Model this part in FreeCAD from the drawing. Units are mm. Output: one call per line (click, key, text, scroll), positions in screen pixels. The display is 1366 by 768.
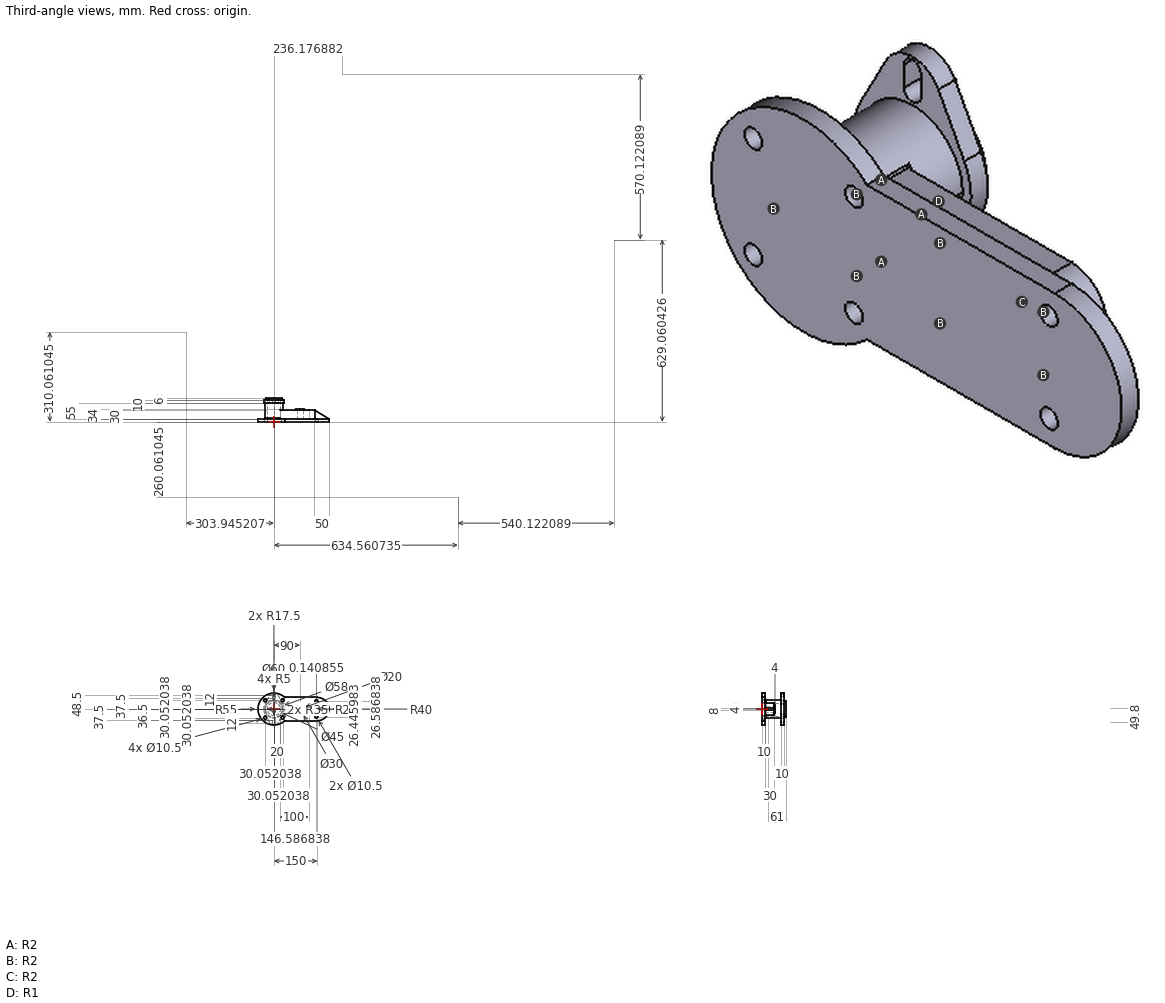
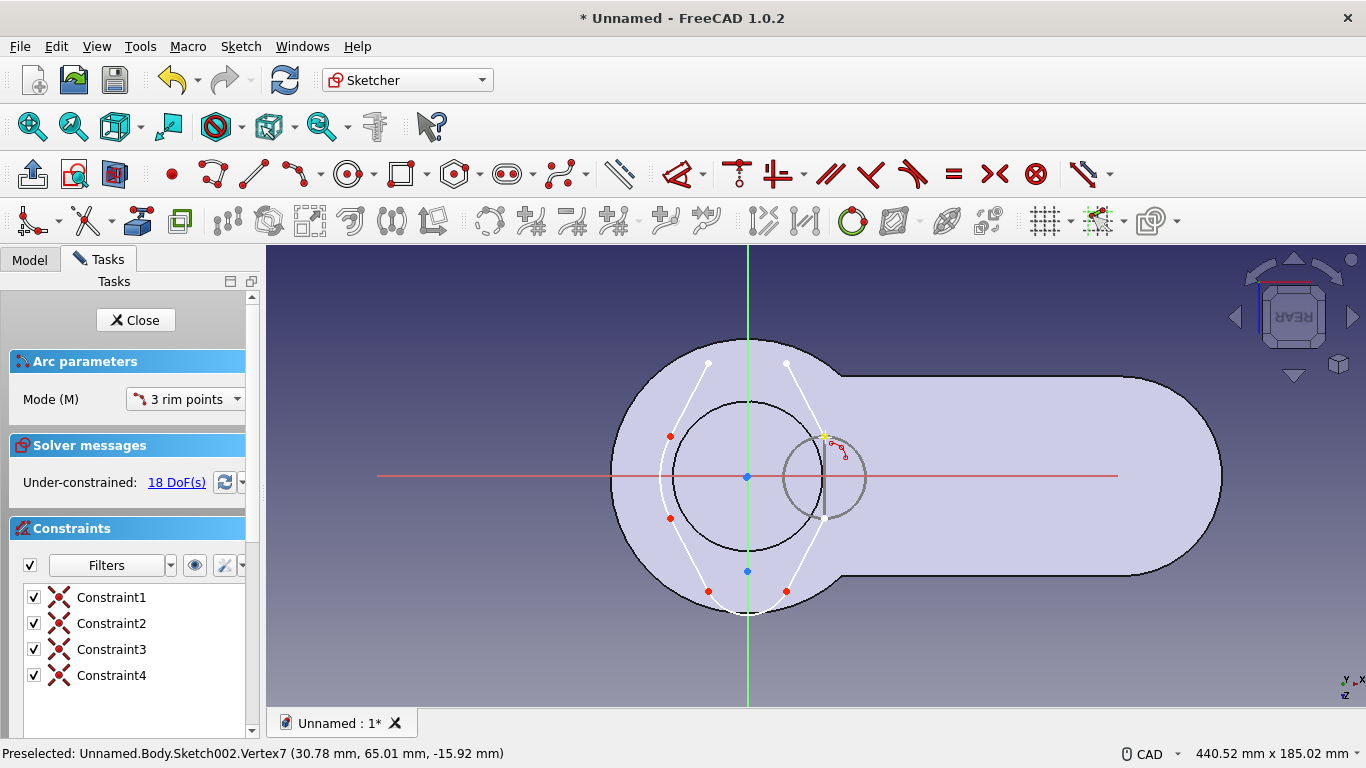
scroll(835, 468, up, 4)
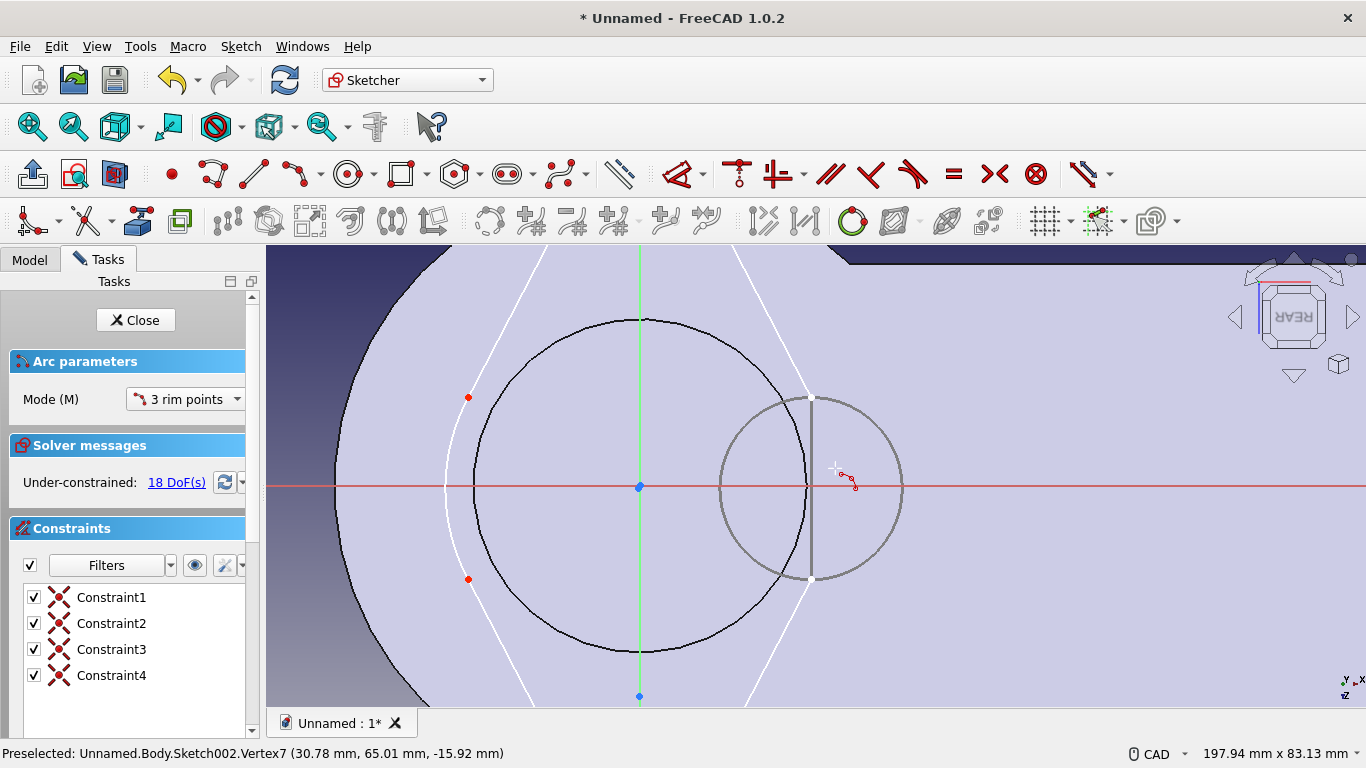
click(834, 467)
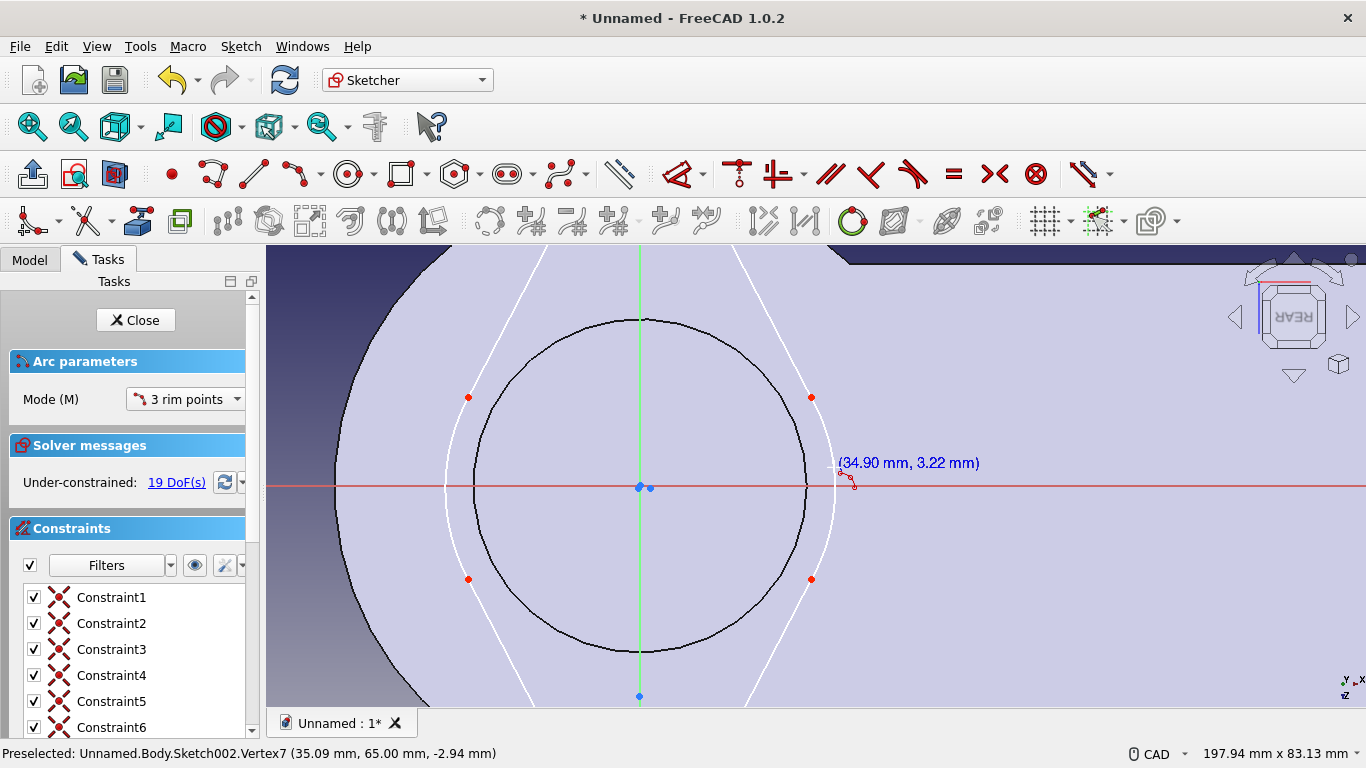
scroll(835, 468, down, 4)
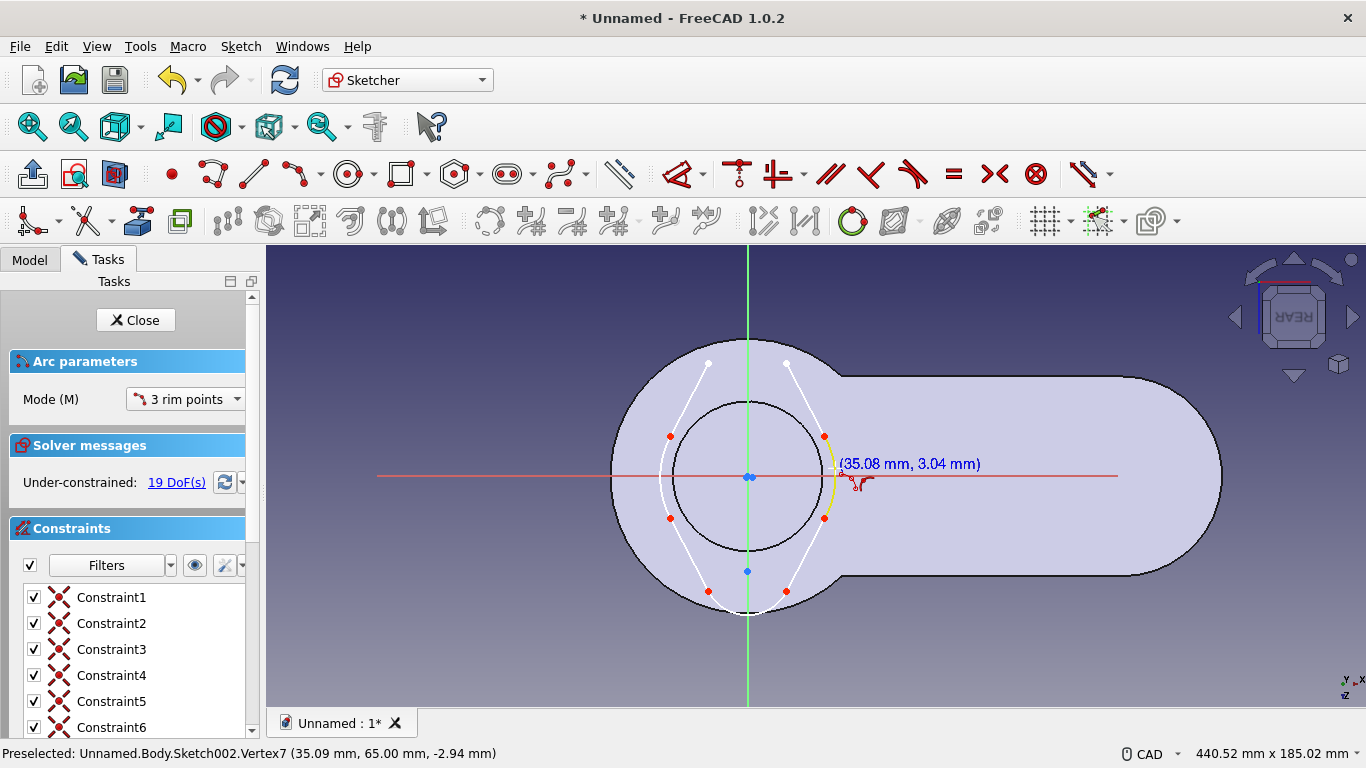
click(787, 364)
click(709, 364)
click(766, 343)
key(Escape)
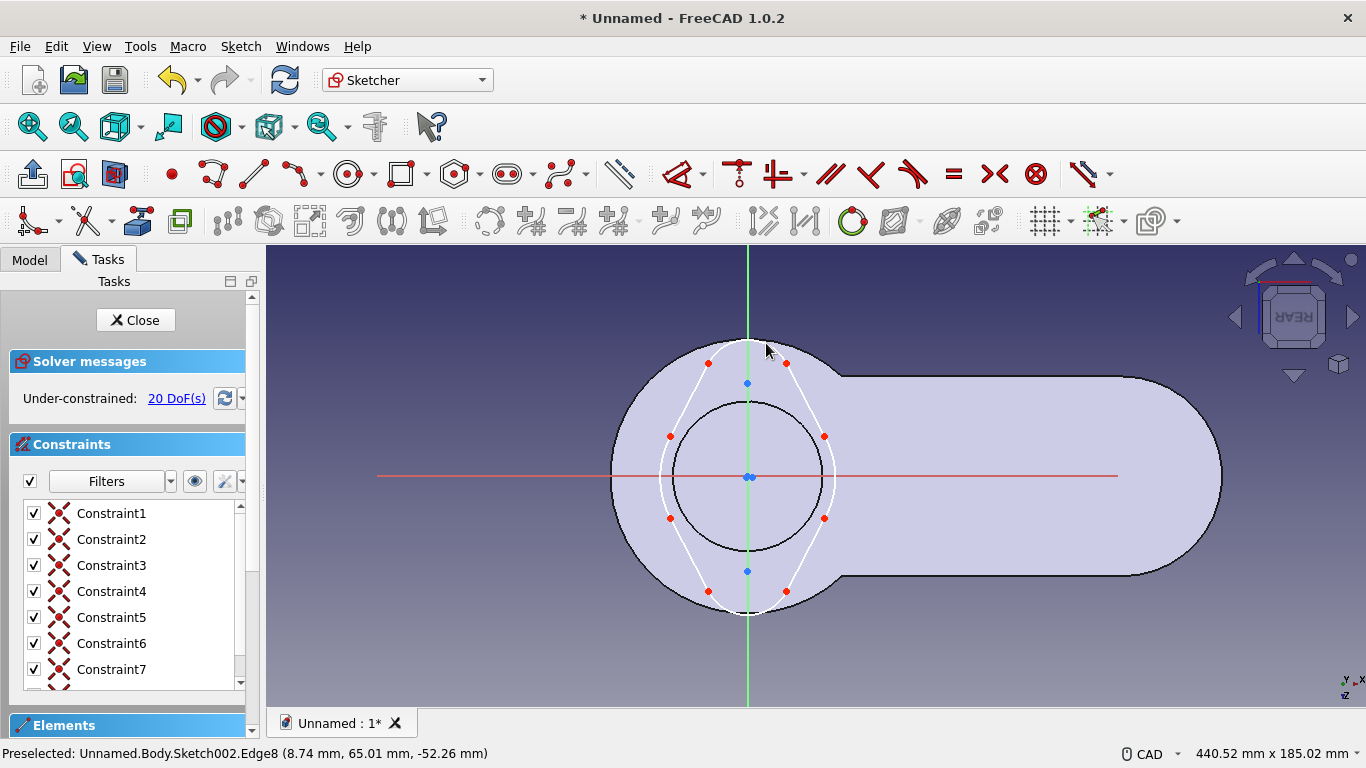
click(697, 385)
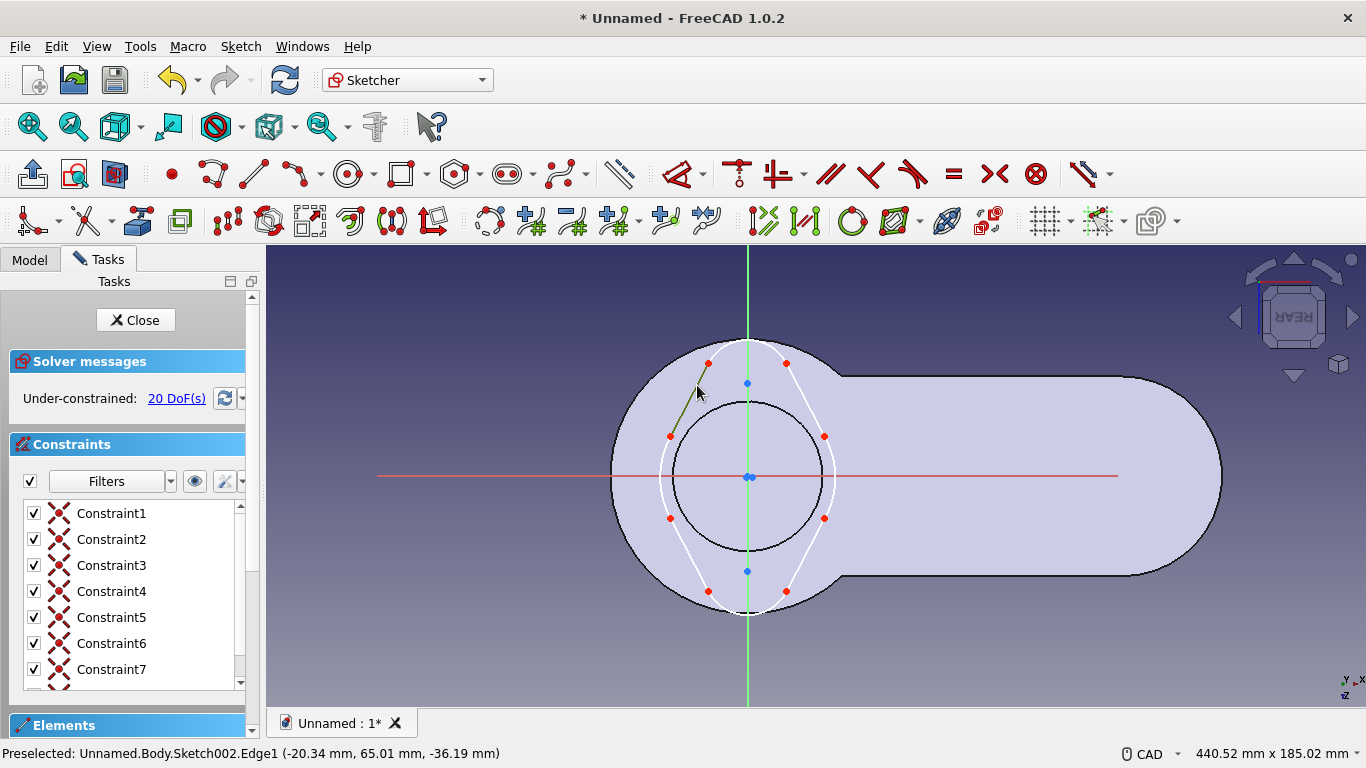
click(662, 461)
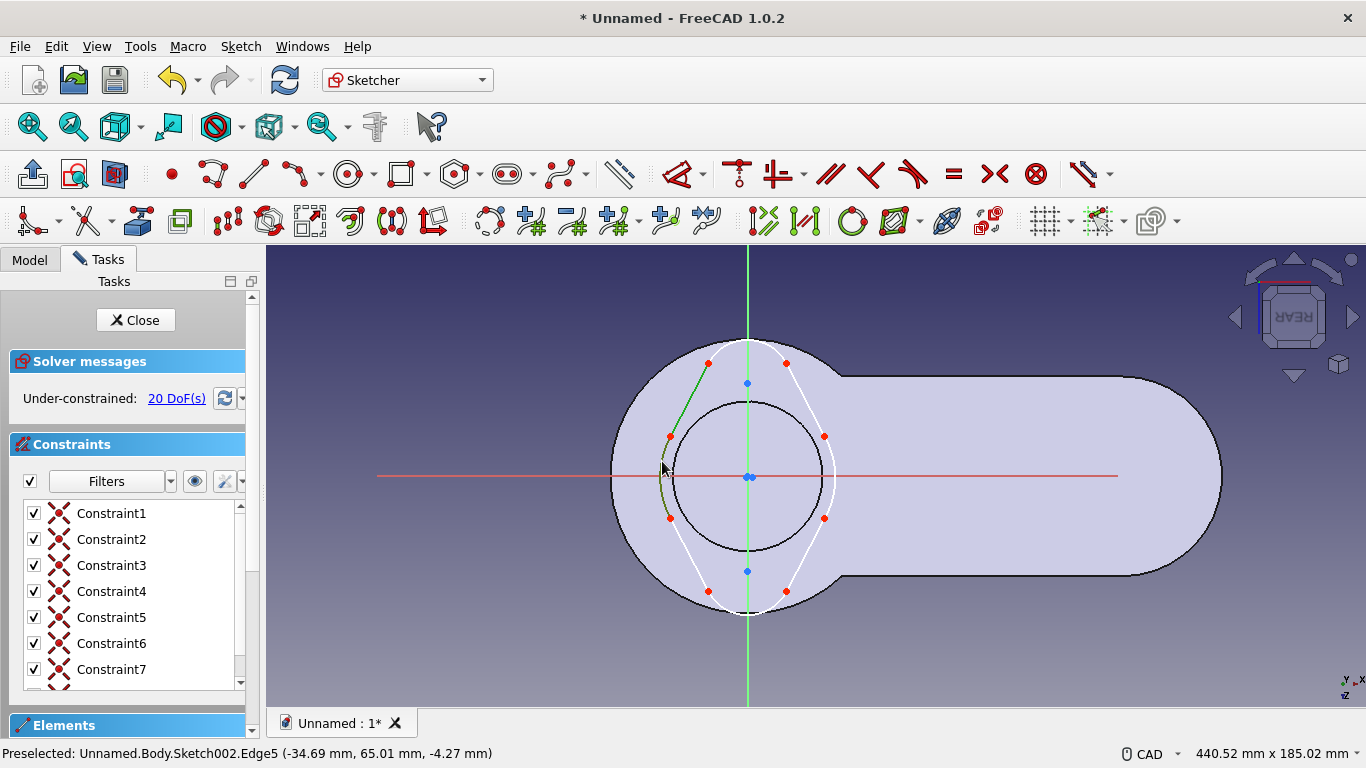
key(t)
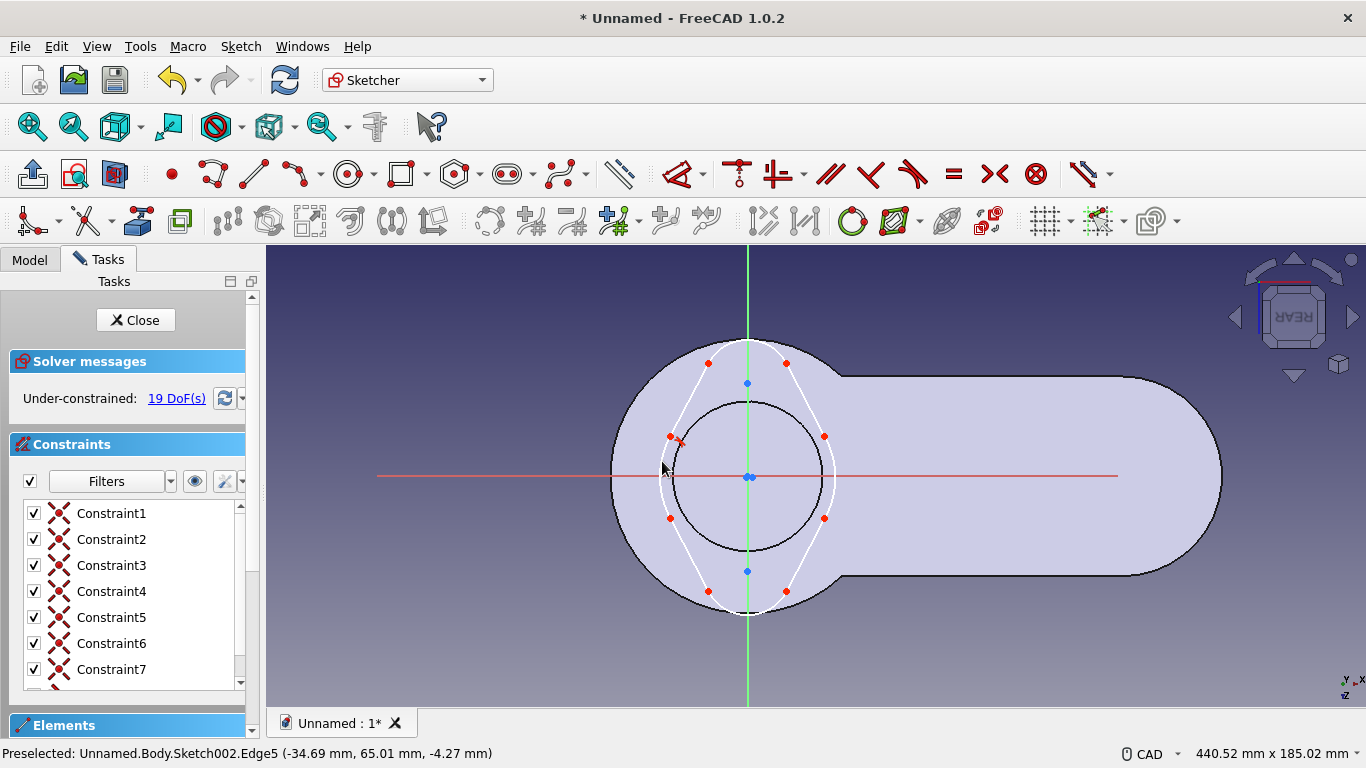
click(697, 385)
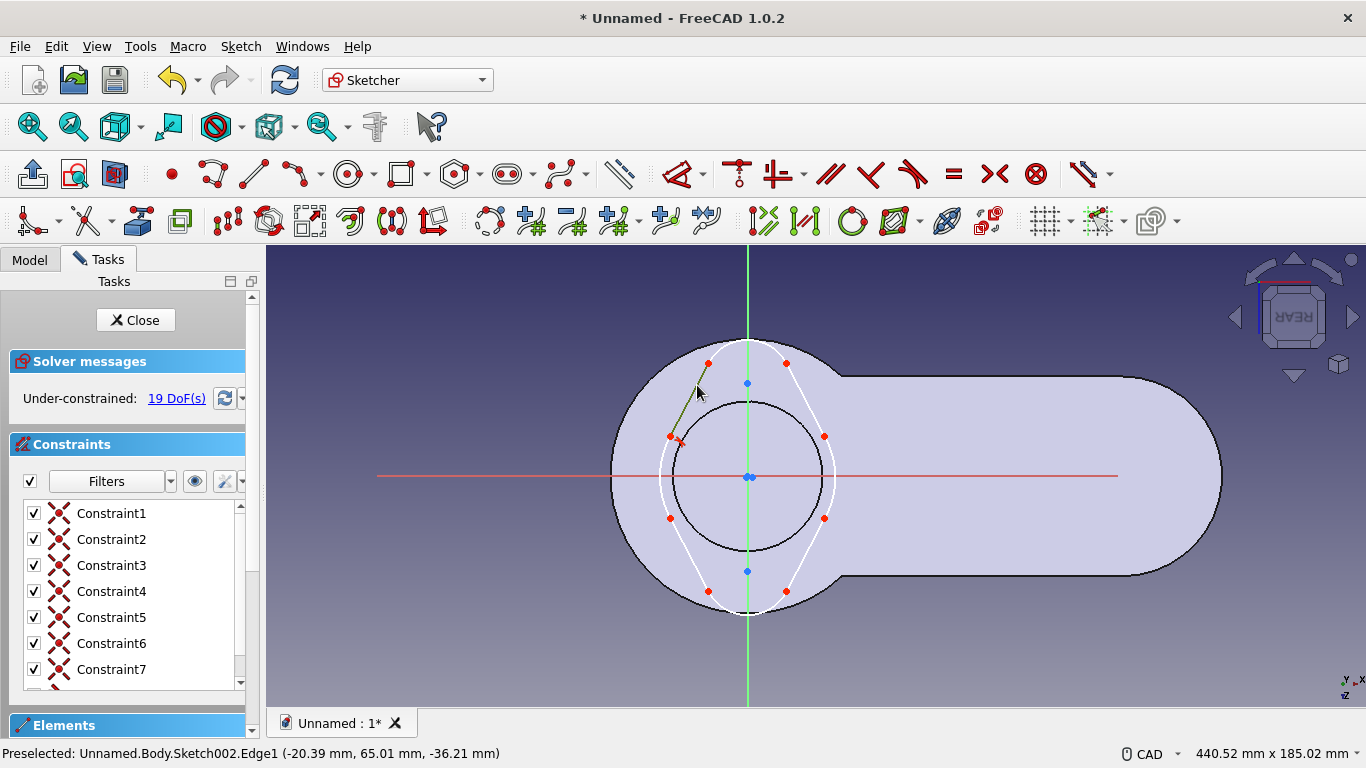
click(766, 344)